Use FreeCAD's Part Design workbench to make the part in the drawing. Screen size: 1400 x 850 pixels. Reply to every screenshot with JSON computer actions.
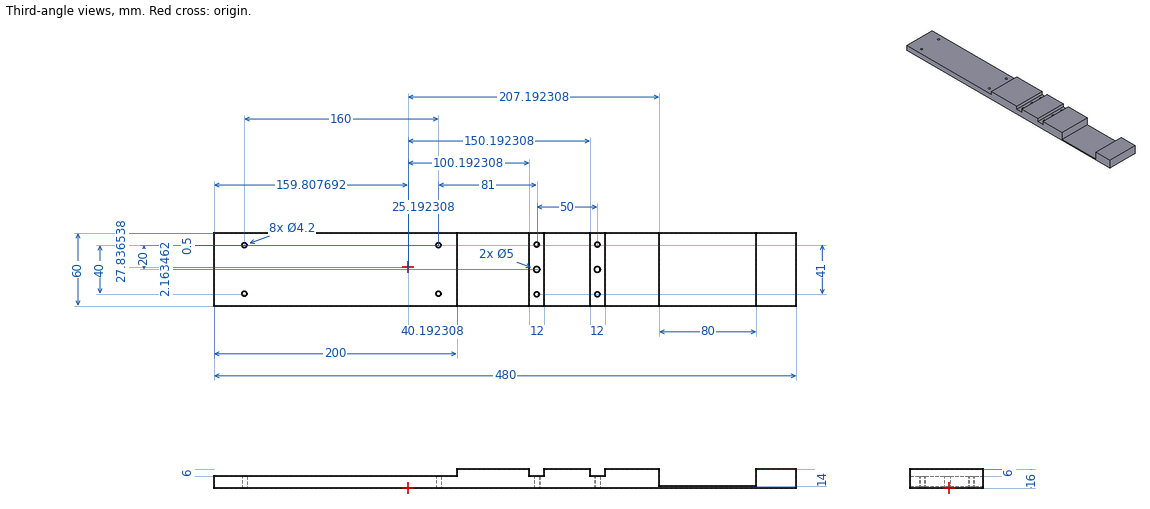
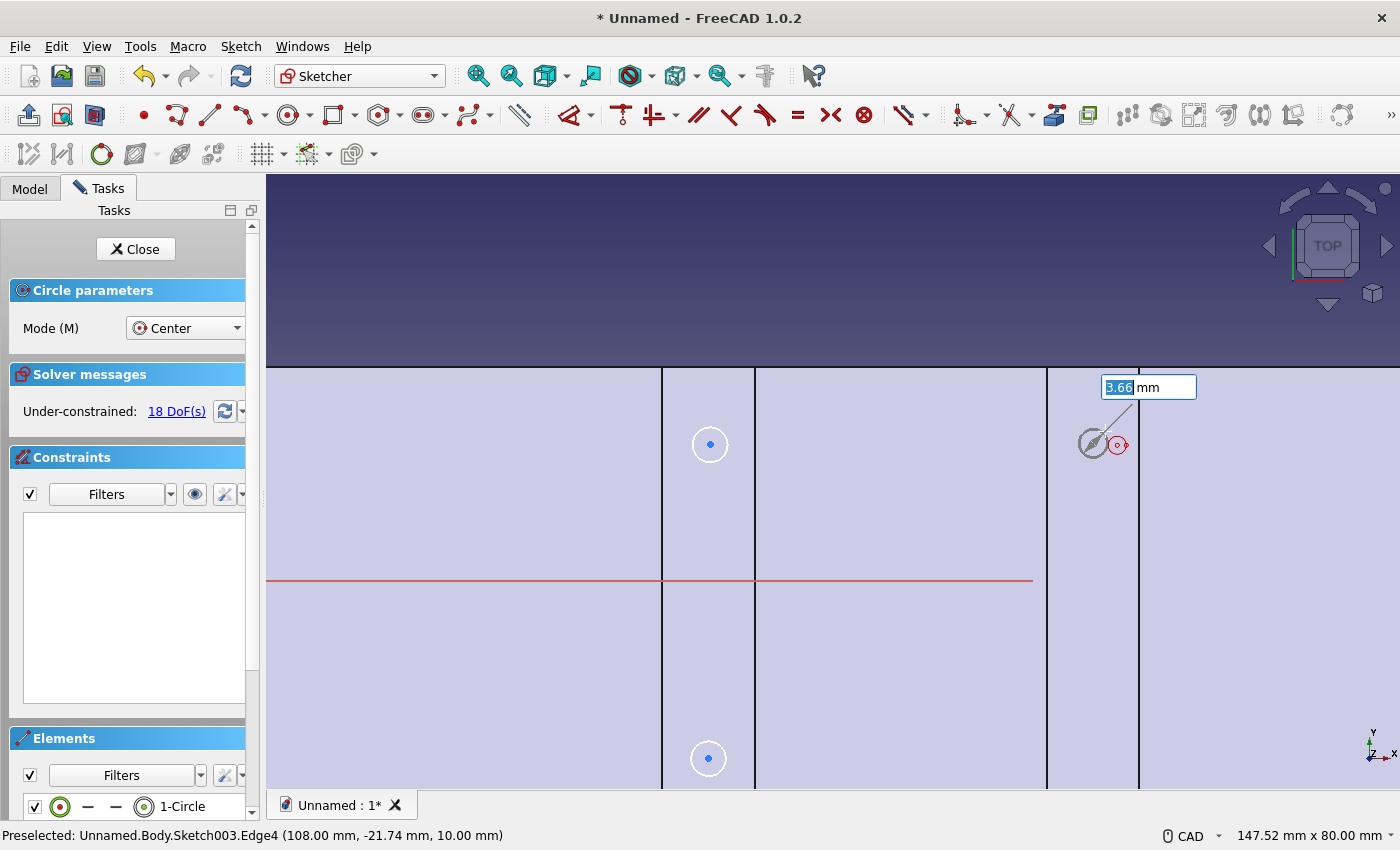
{"action": "left_click", "coordinate": [1104, 429]}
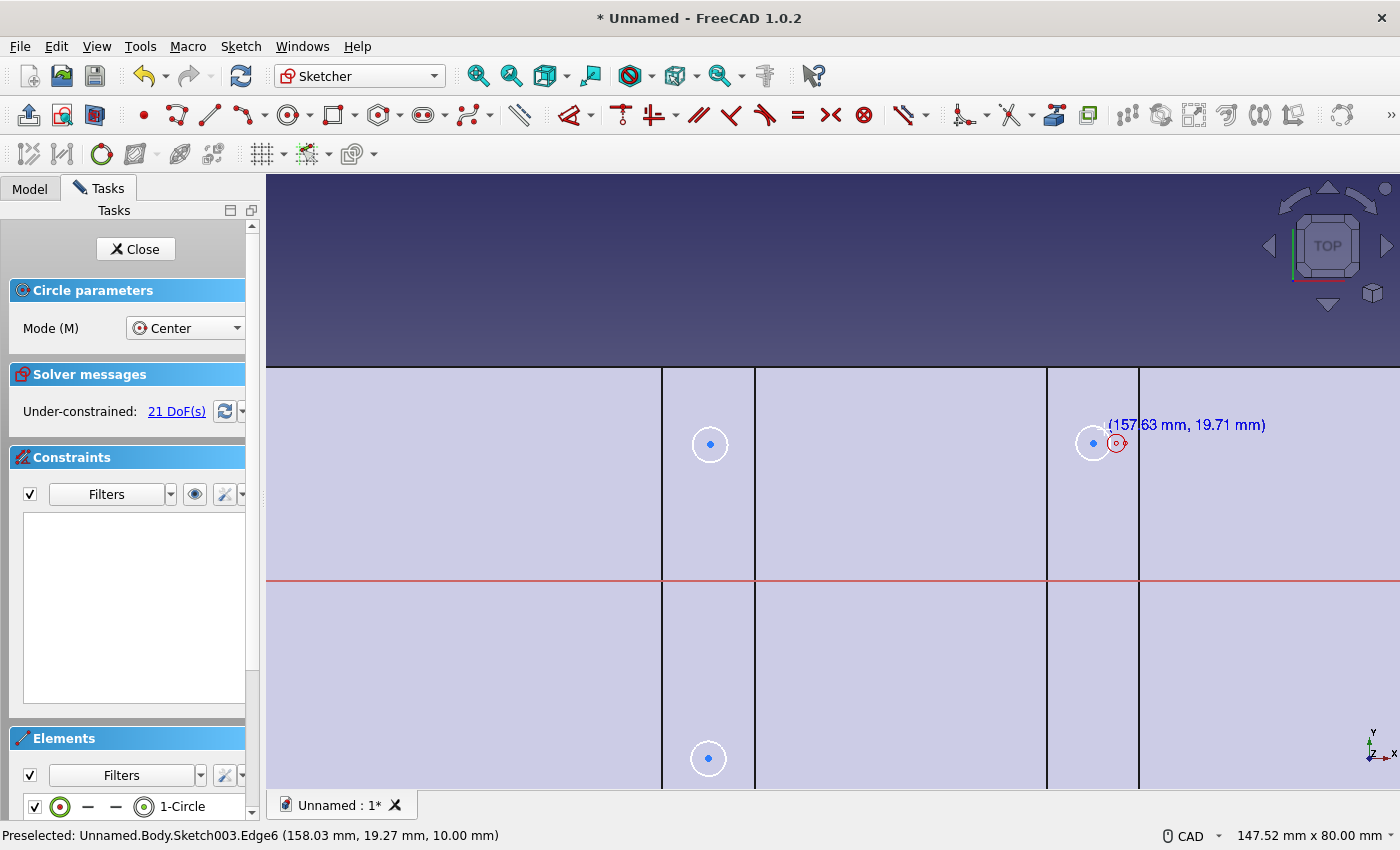
{"action": "scroll", "coordinate": [1093, 756], "scroll_direction": "up", "scroll_amount": 2}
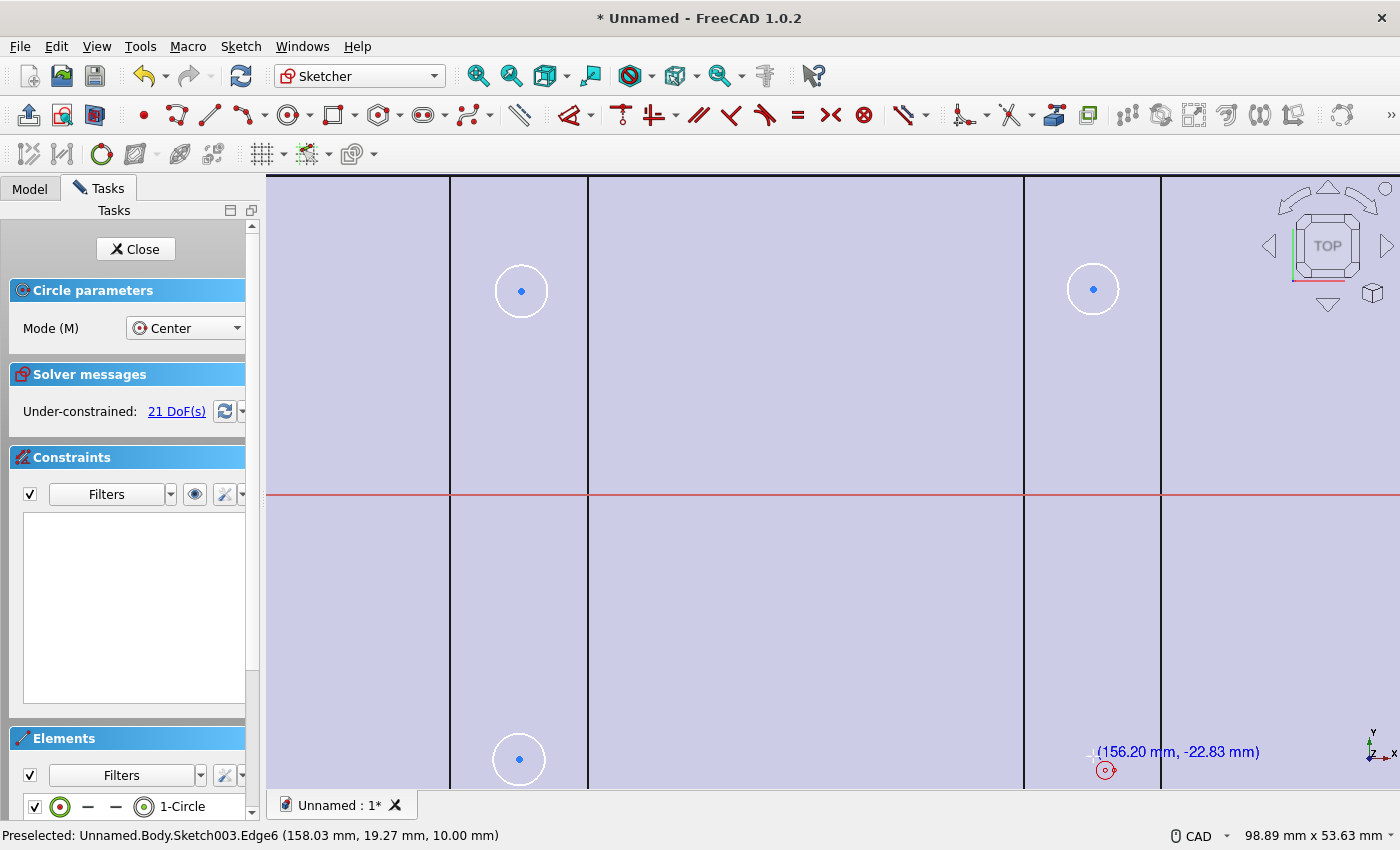
{"action": "scroll", "coordinate": [1103, 472], "scroll_direction": "down", "scroll_amount": 8}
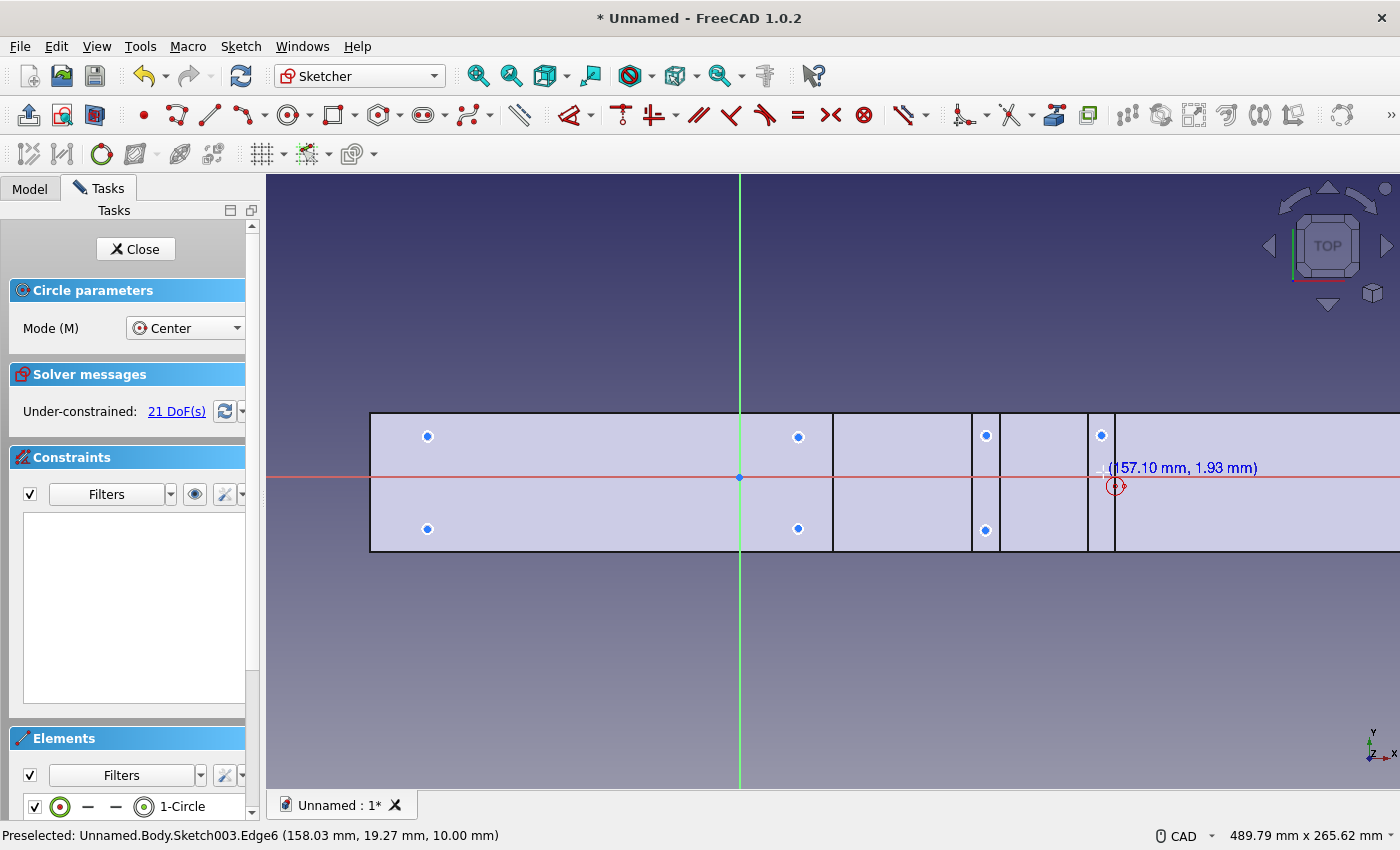
{"action": "left_click", "coordinate": [1101, 530]}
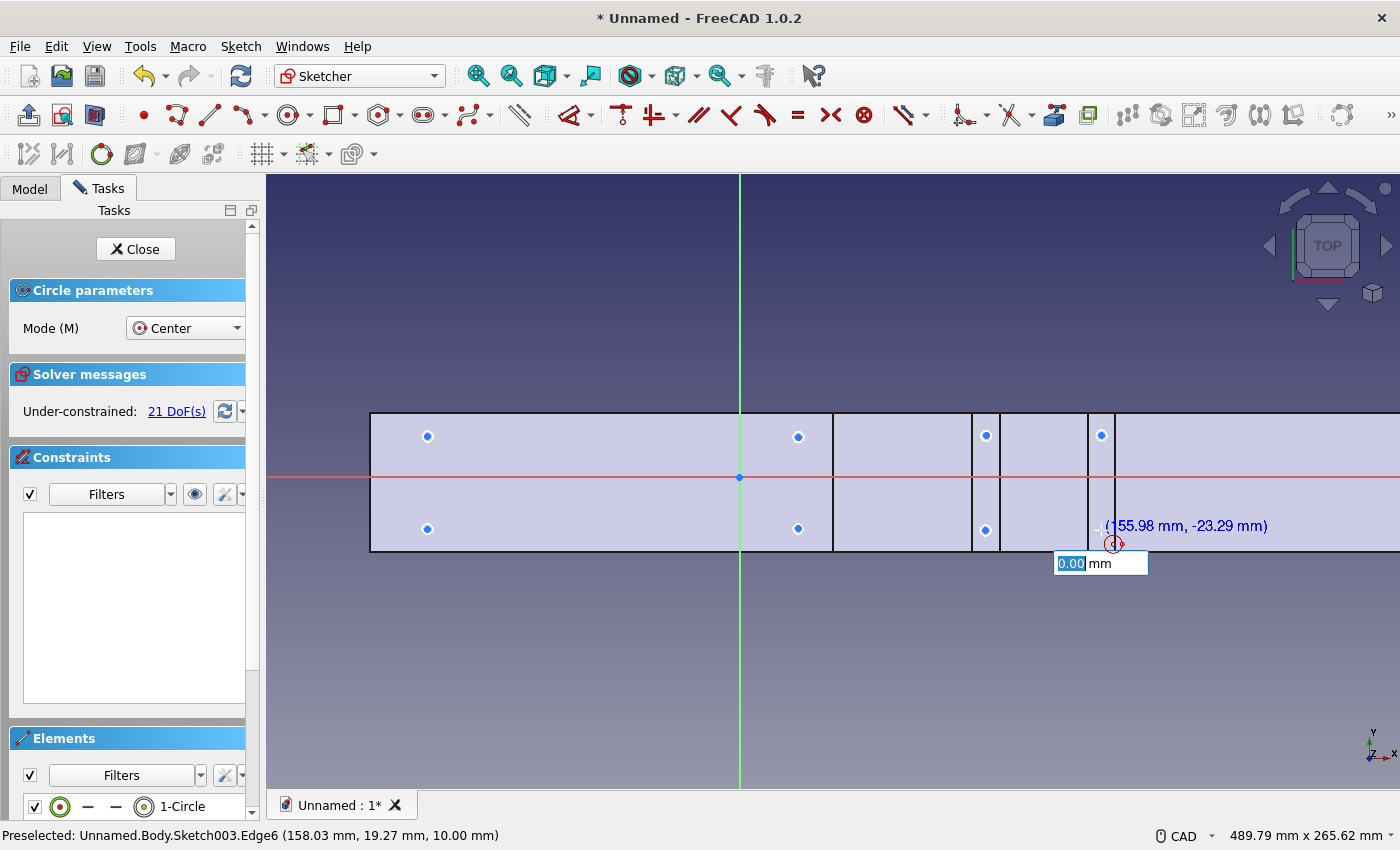
{"action": "scroll", "coordinate": [1105, 526], "scroll_direction": "up", "scroll_amount": 6}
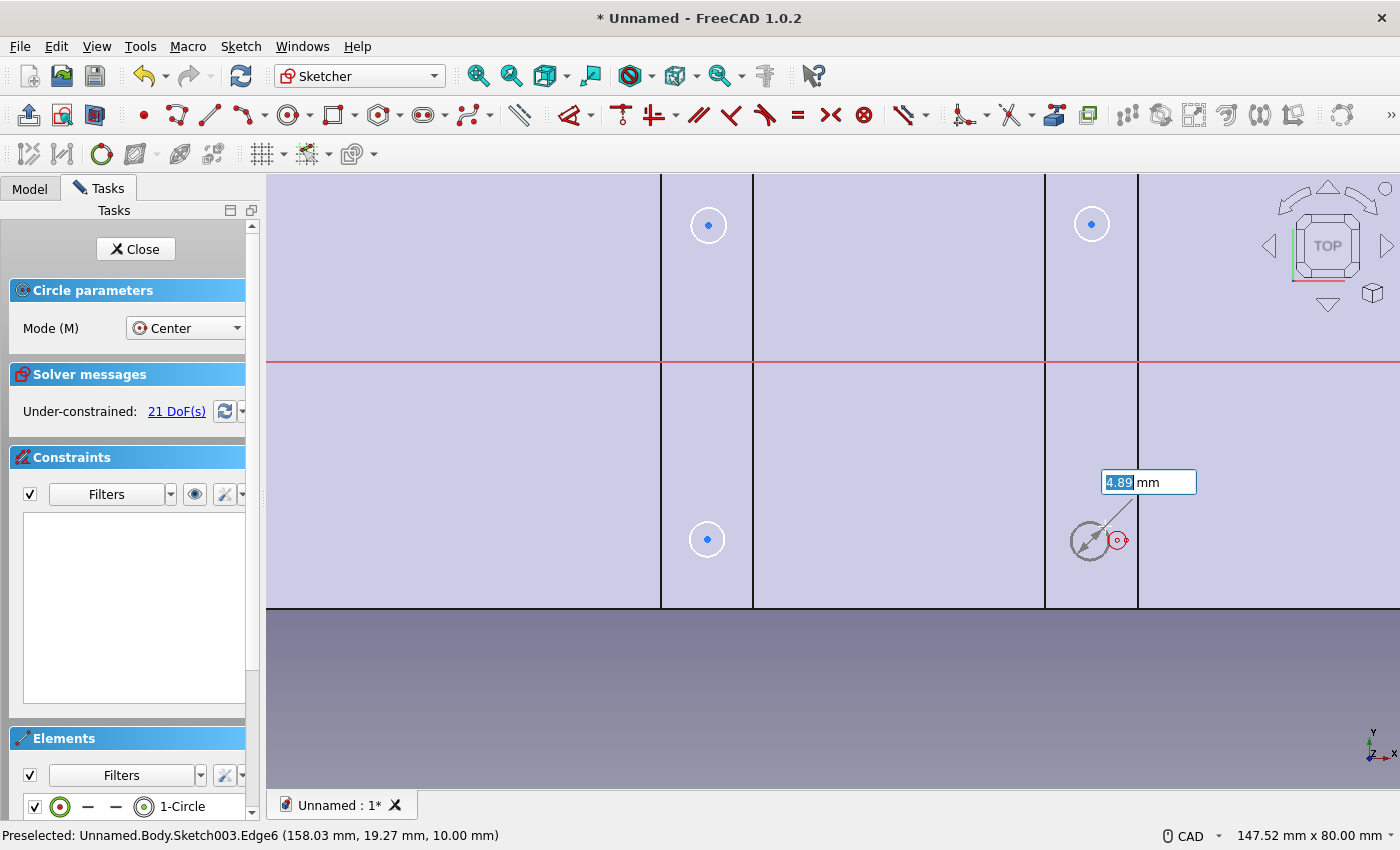
{"action": "left_click", "coordinate": [1103, 525]}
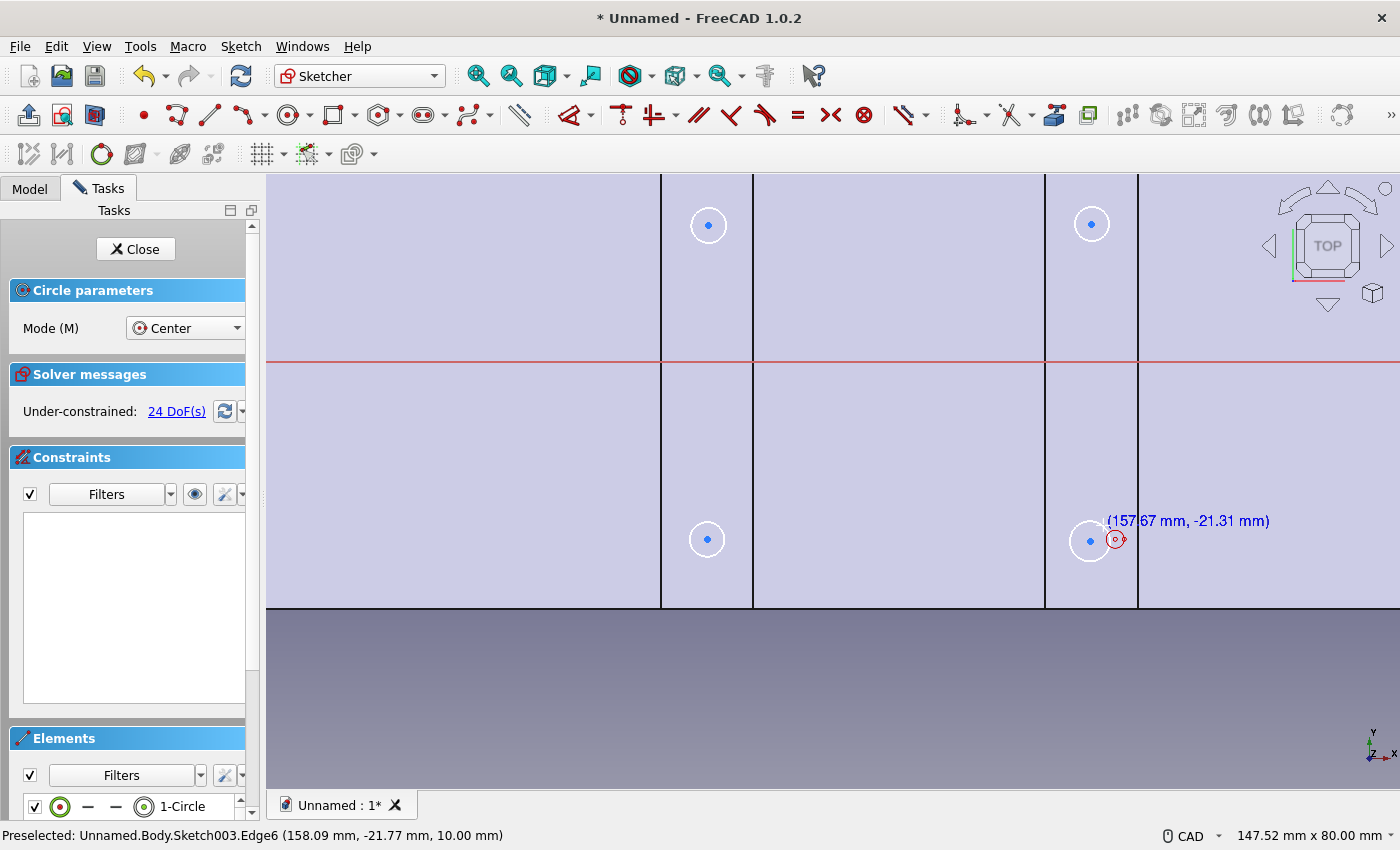
{"action": "left_click", "coordinate": [707, 379]}
{"action": "left_click", "coordinate": [721, 392]}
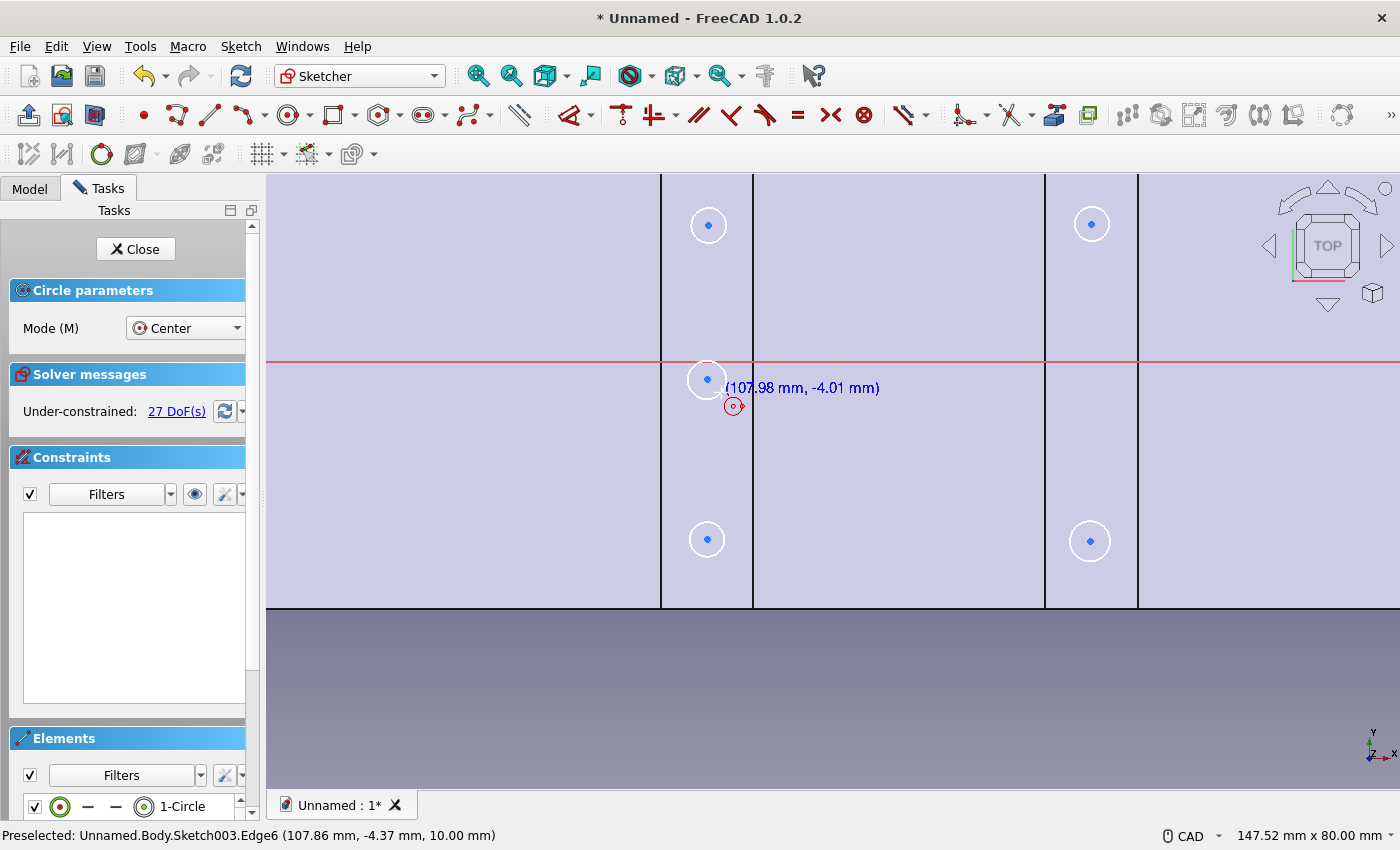
{"action": "left_click", "coordinate": [1092, 379]}
{"action": "left_click", "coordinate": [1105, 392]}
{"action": "key", "text": "Escape"}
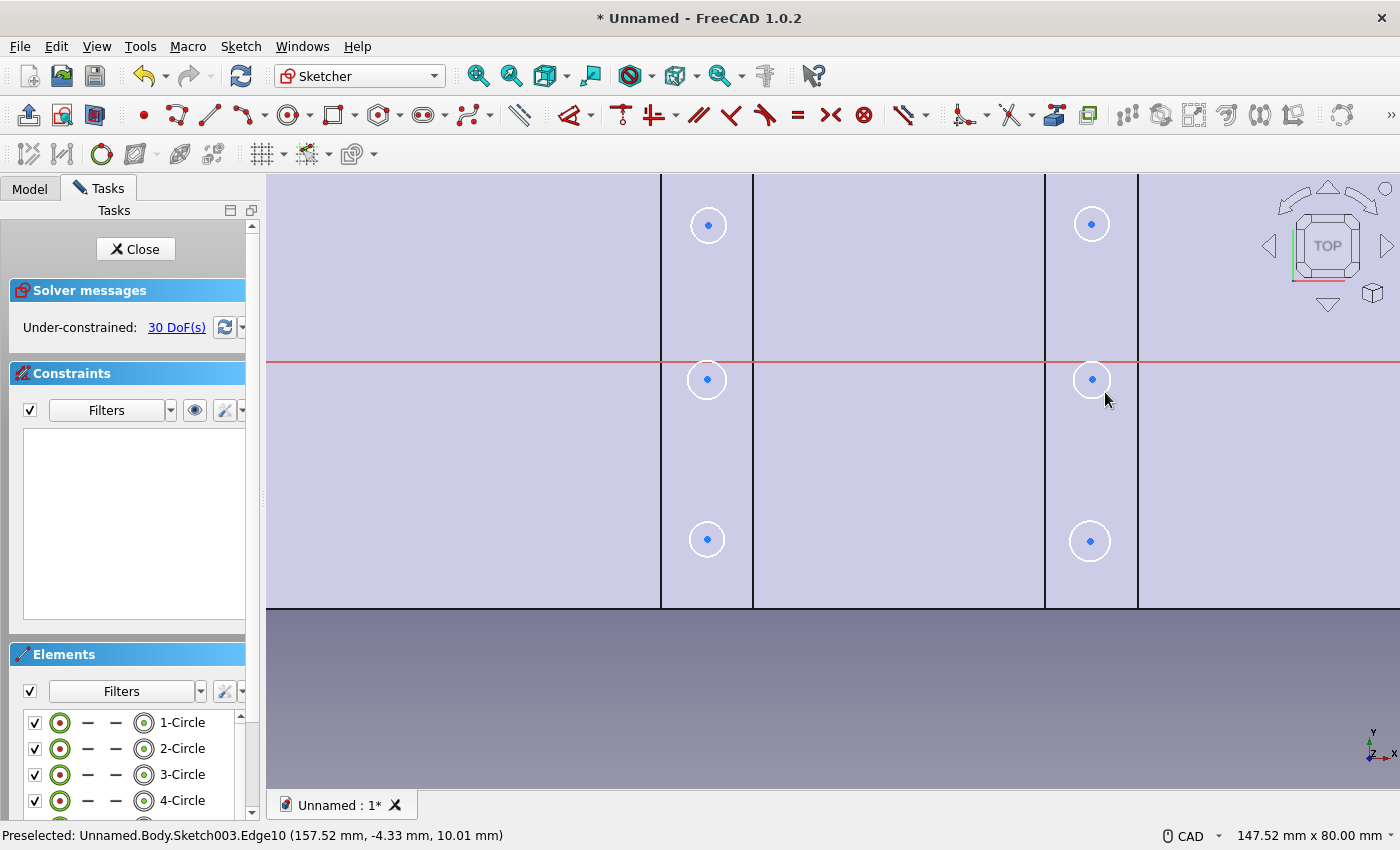
{"action": "scroll", "coordinate": [1105, 526], "scroll_direction": "down", "scroll_amount": 6}